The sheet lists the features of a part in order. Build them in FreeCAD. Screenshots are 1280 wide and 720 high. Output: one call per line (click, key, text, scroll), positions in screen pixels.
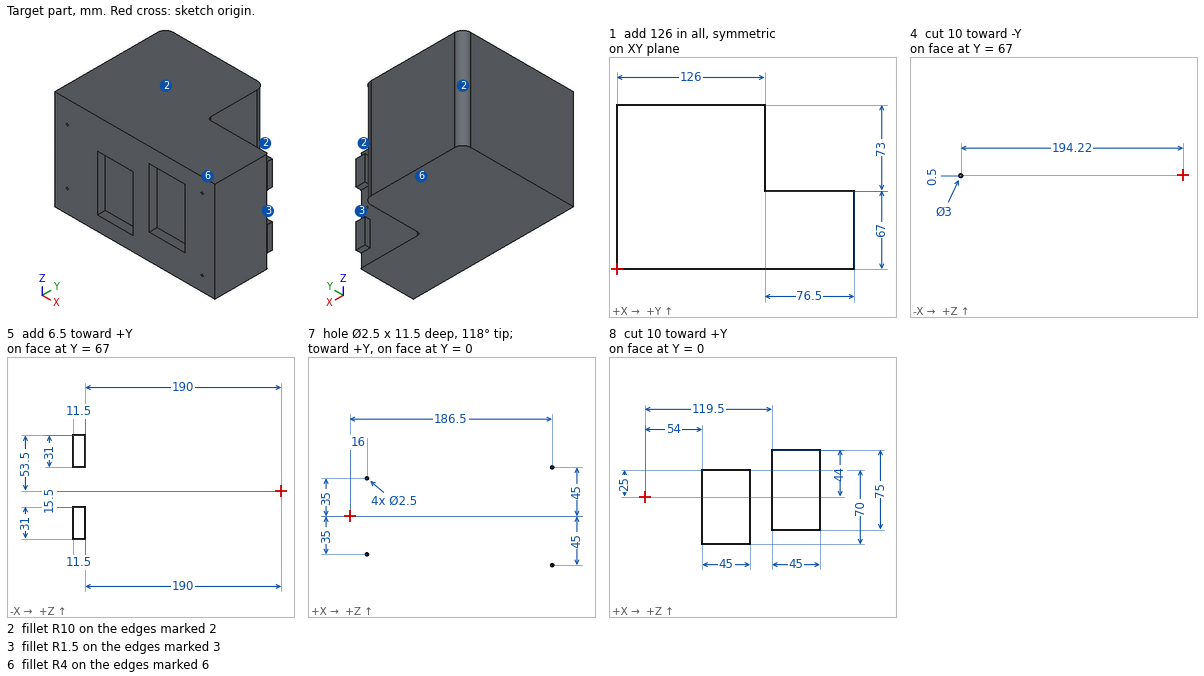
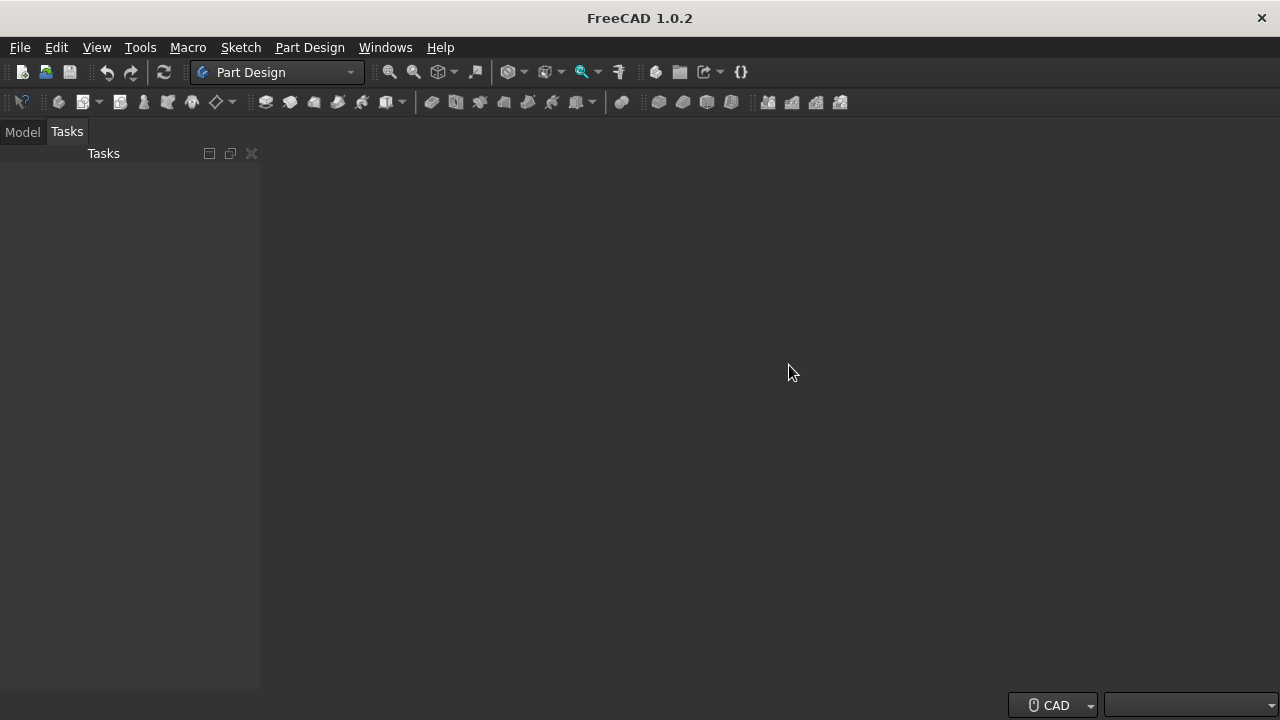
key(ctrl+n)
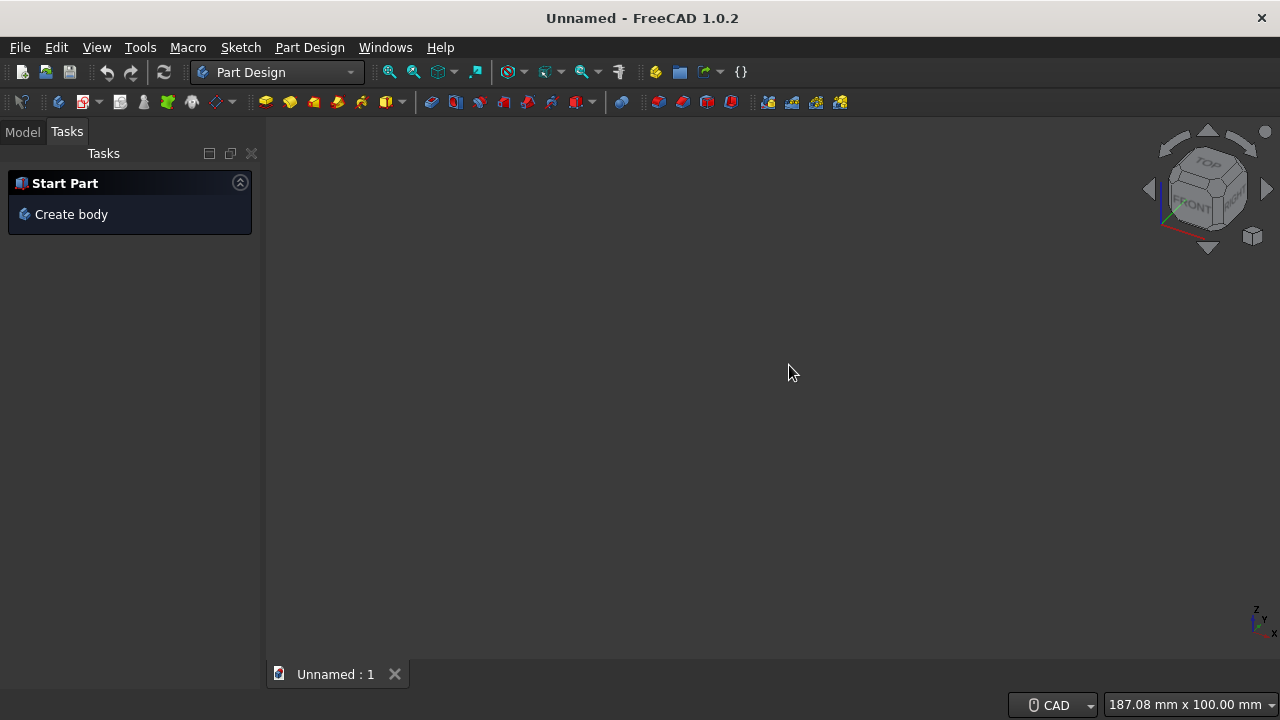
click(84, 102)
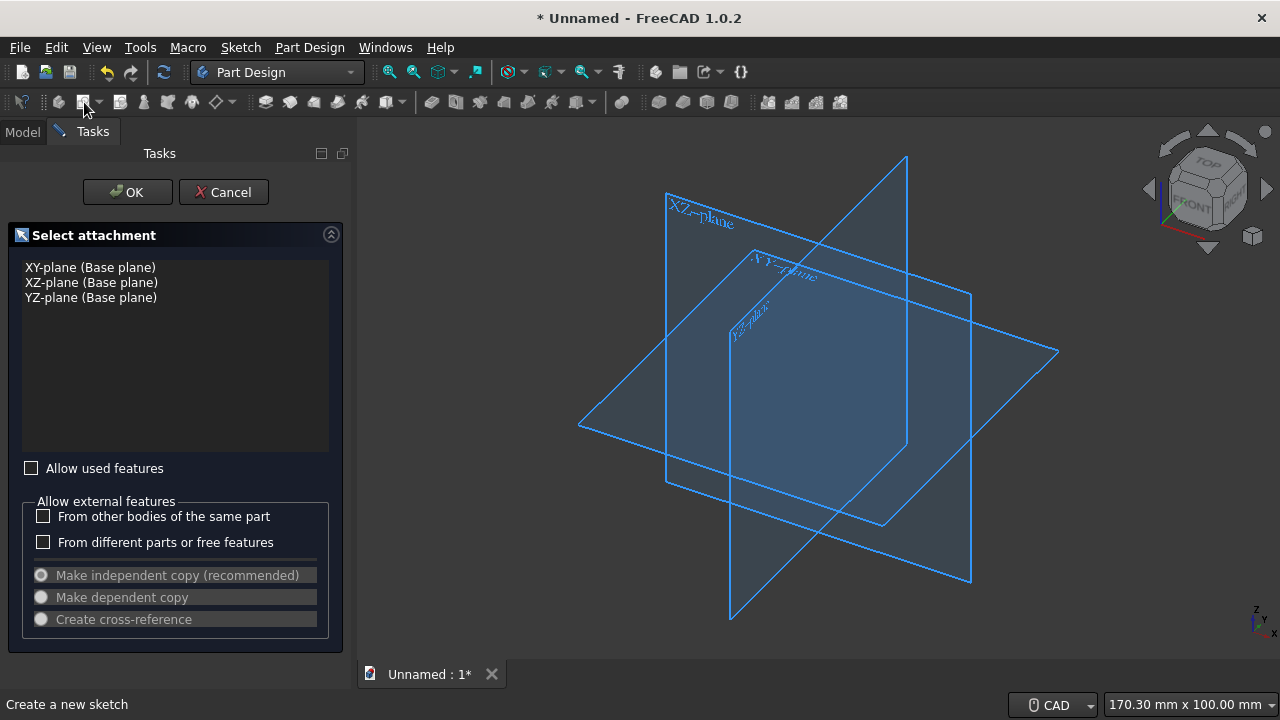
click(82, 268)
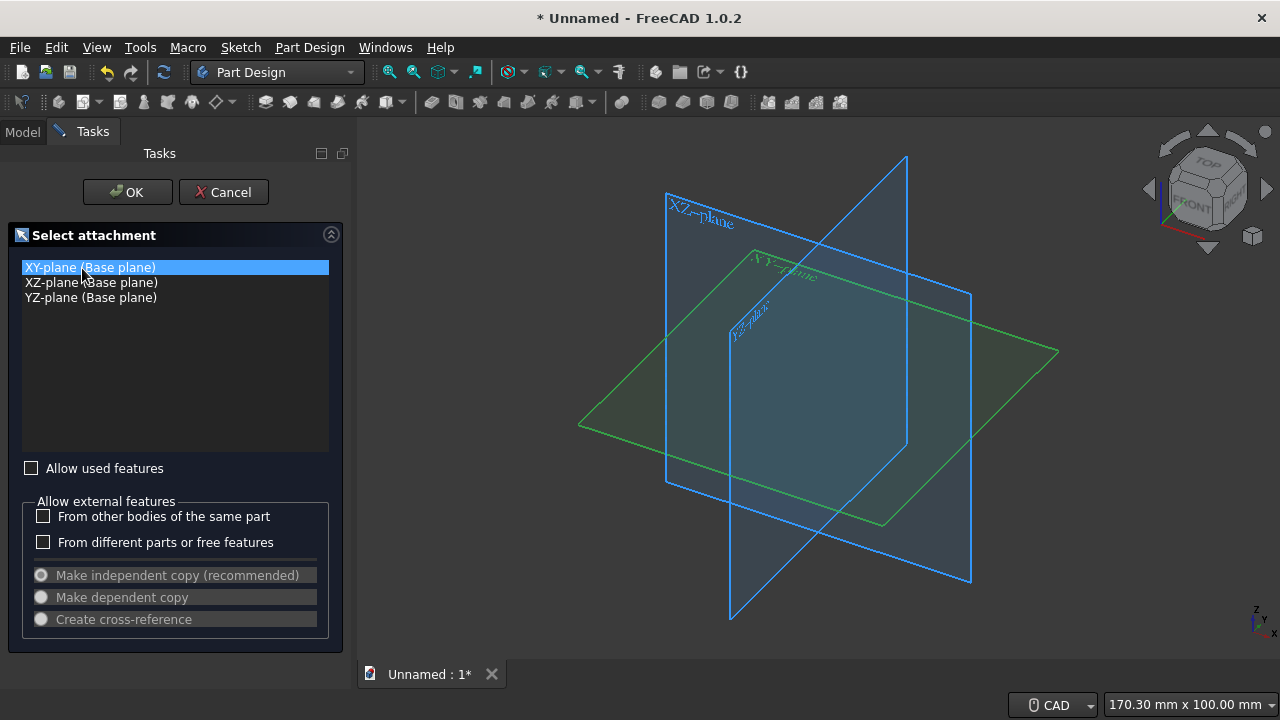
click(128, 192)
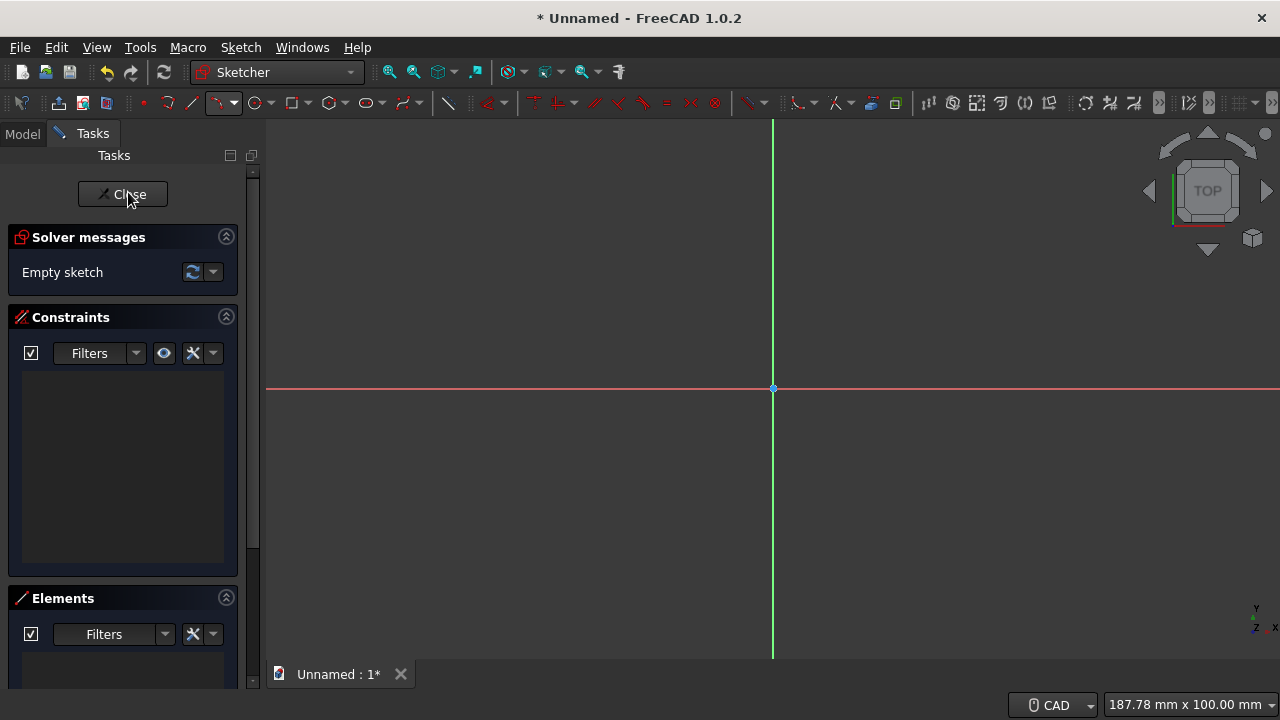
scroll(294, 631, down, 4)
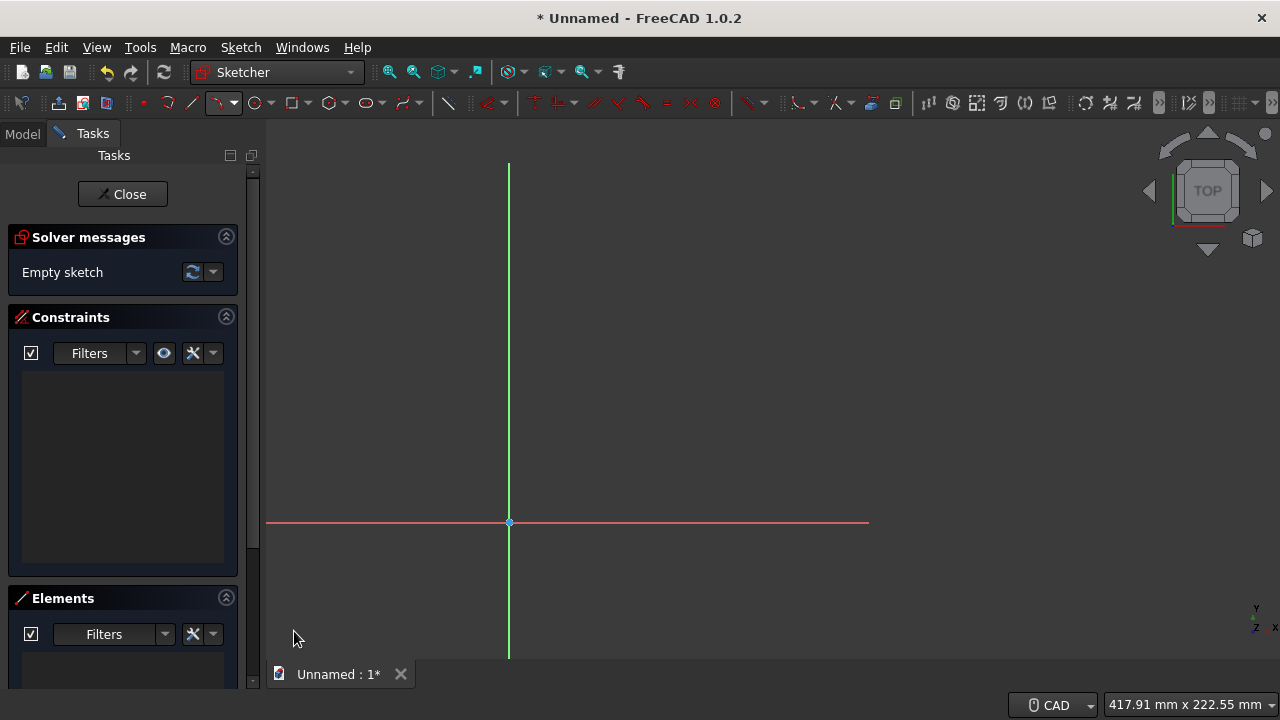
key(g)
key(m)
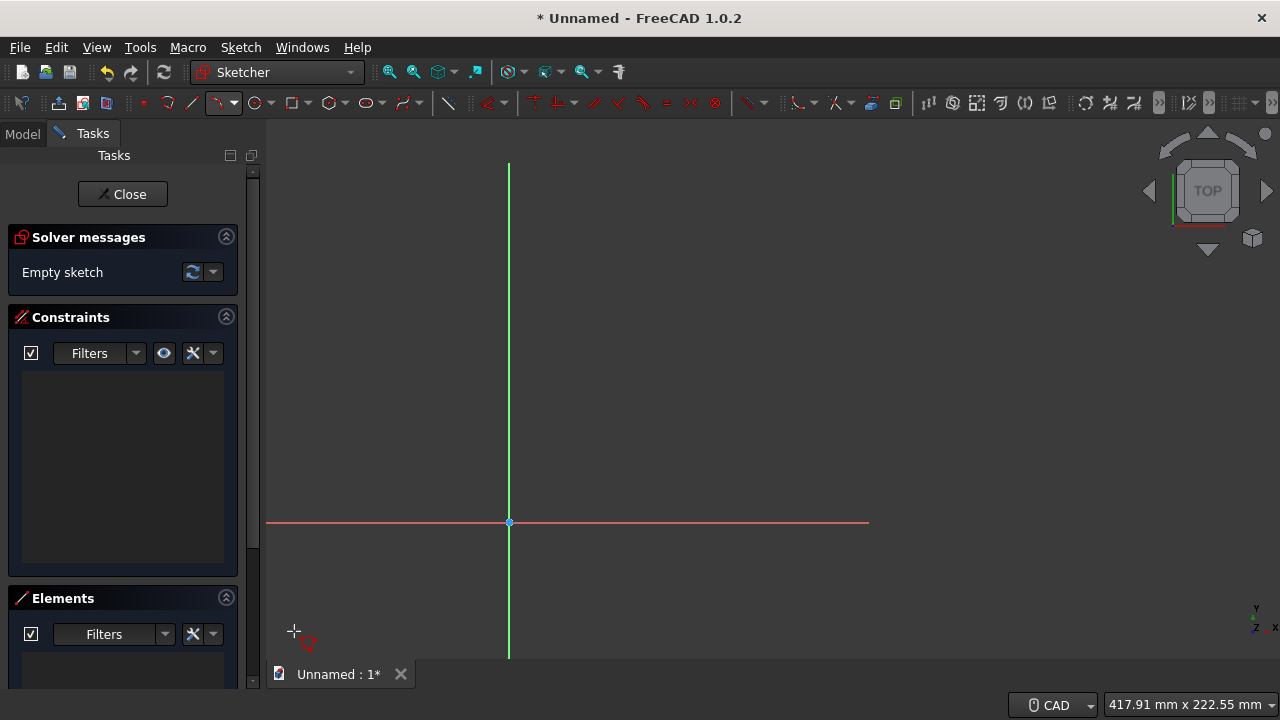
click(509, 523)
click(1001, 514)
click(1001, 360)
click(815, 360)
click(815, 183)
click(518, 183)
click(509, 523)
key(Escape)
key(Escape)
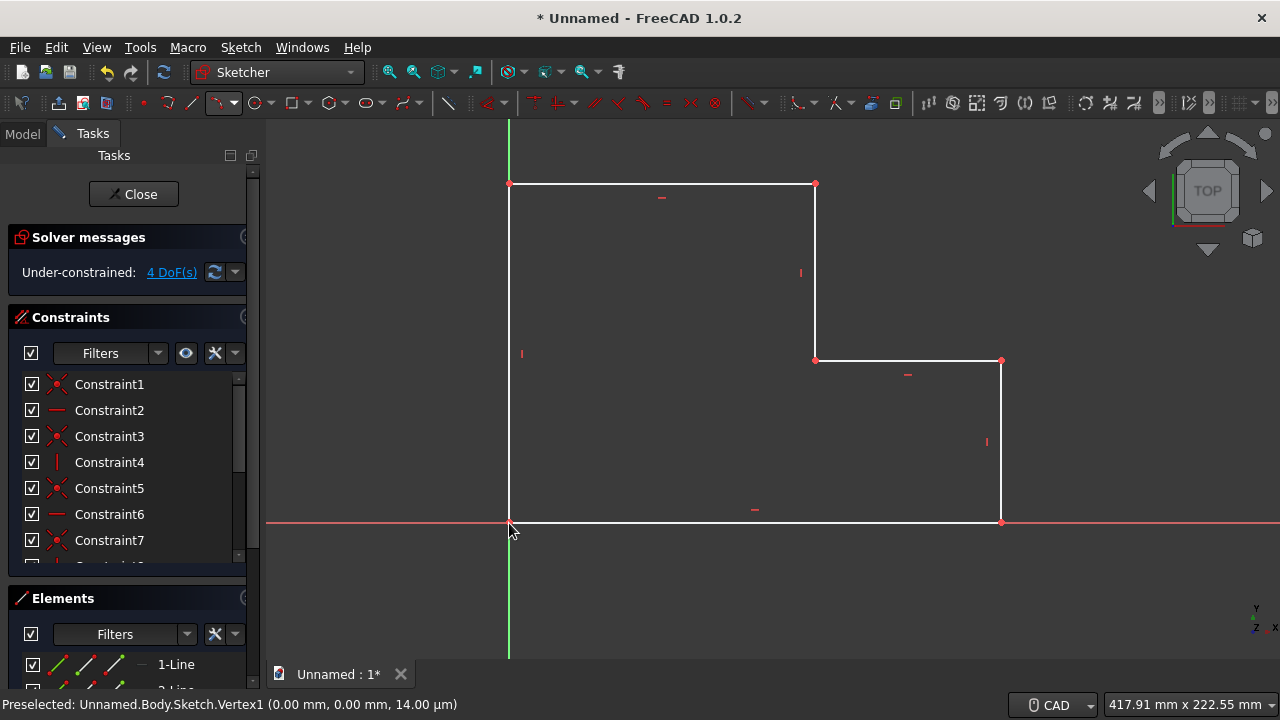
key(d)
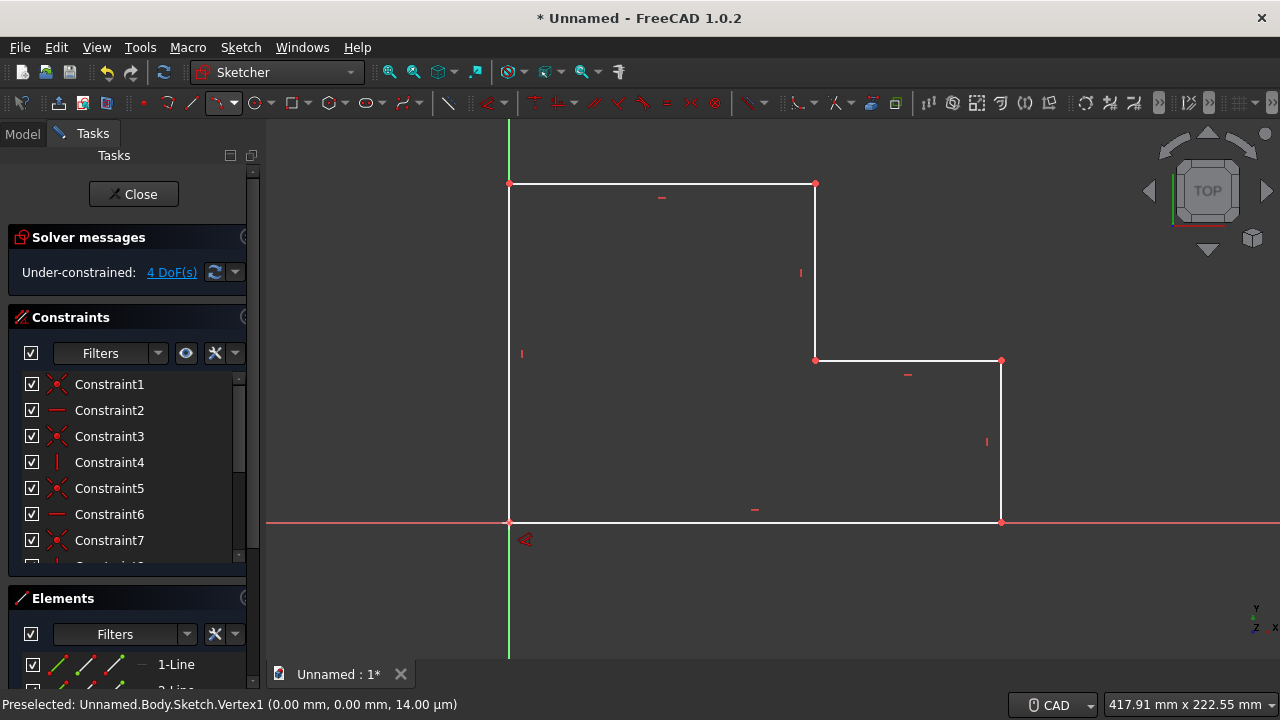
click(1001, 474)
click(1035, 442)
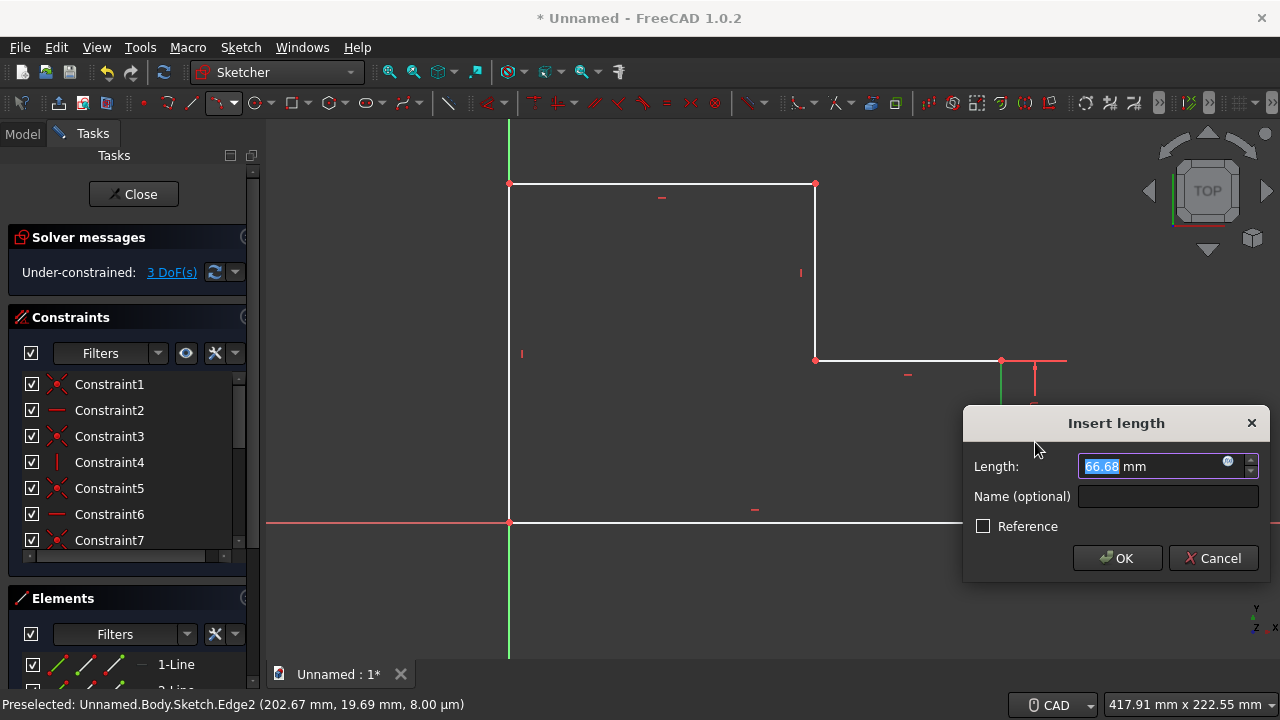
text(67)
key(Return)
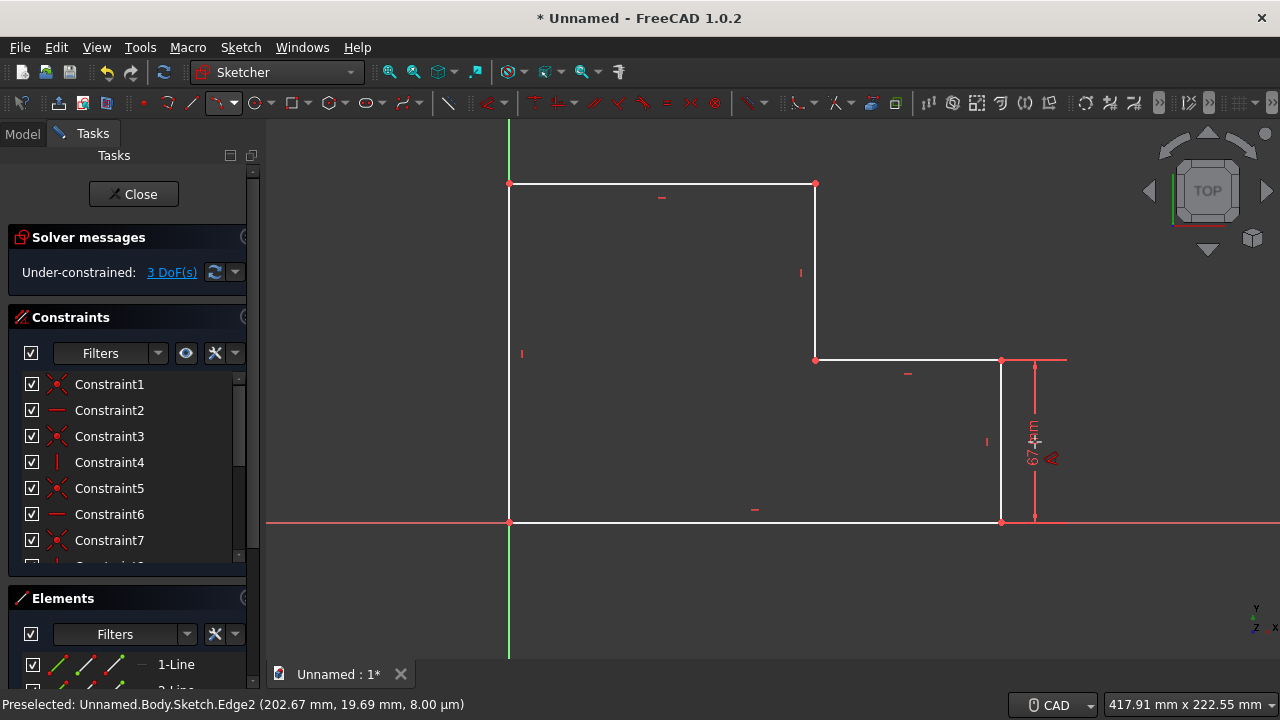
click(815, 307)
click(849, 272)